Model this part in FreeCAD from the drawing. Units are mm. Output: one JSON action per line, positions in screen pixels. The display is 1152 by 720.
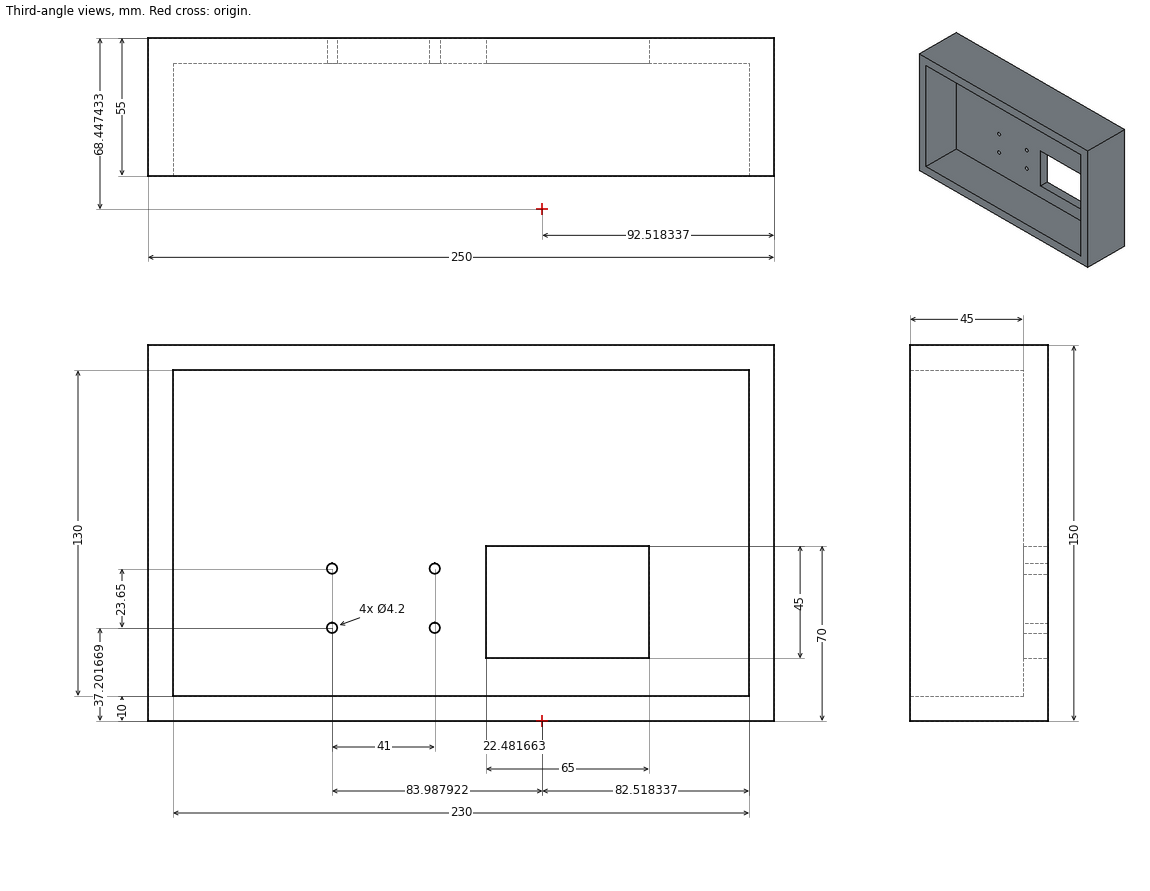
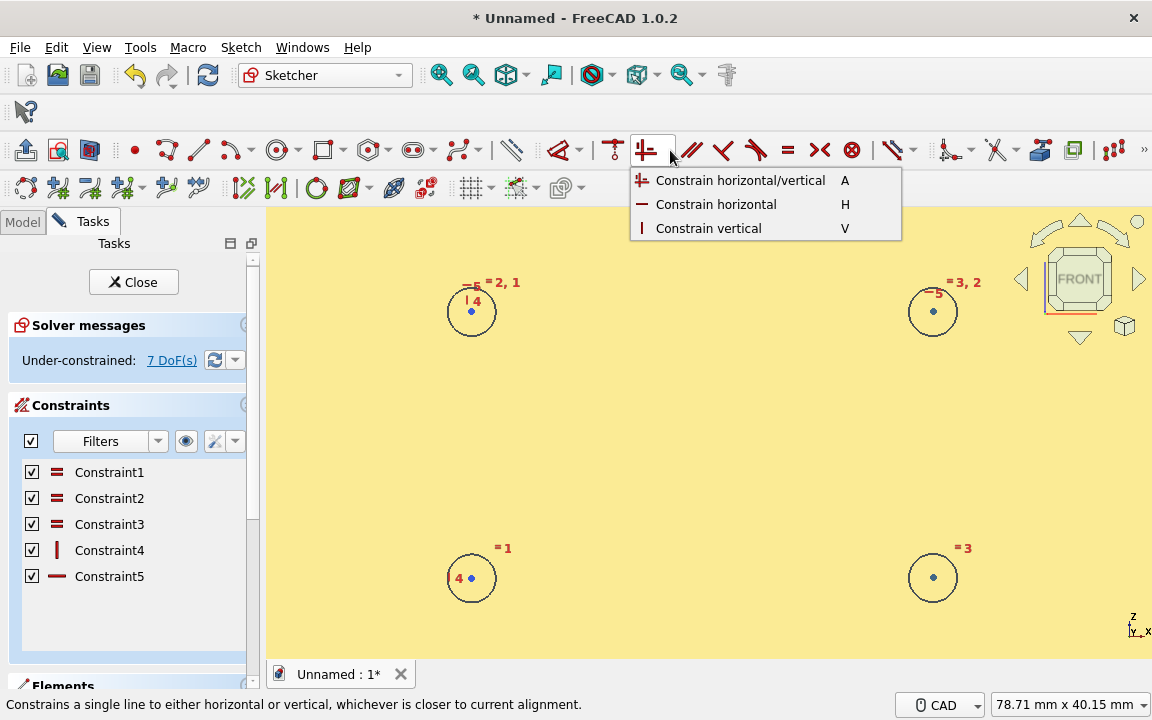
{"action": "left_click", "coordinate": [766, 228]}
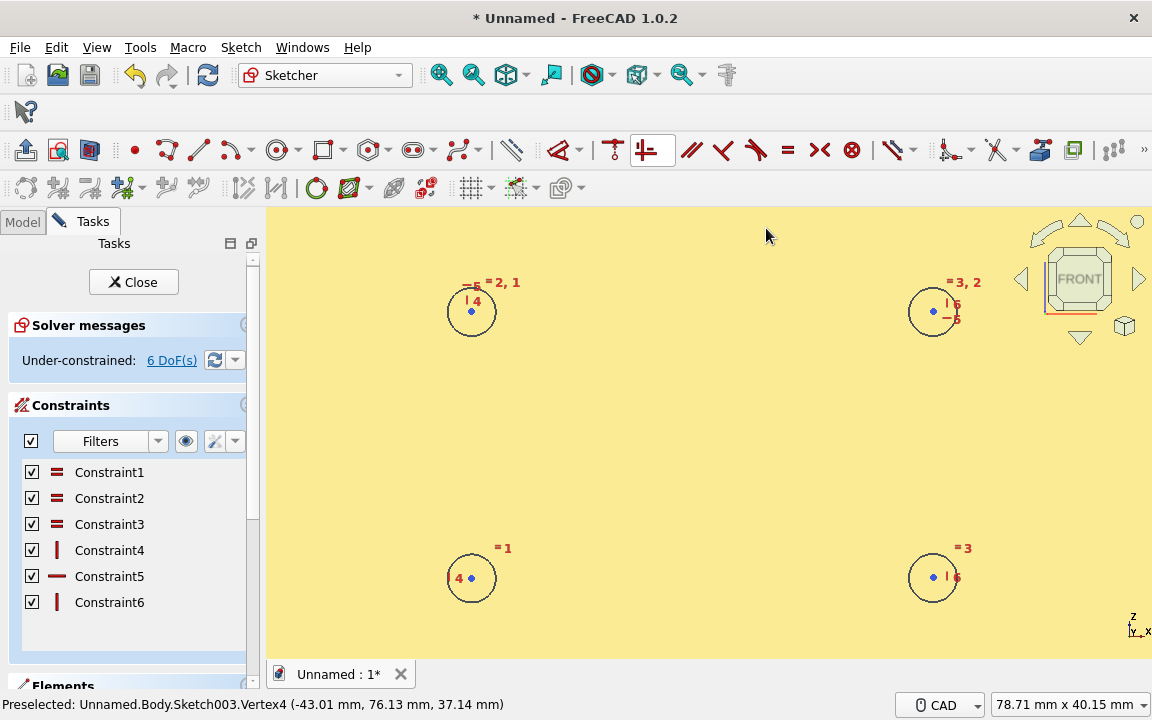
{"action": "left_click", "coordinate": [472, 578]}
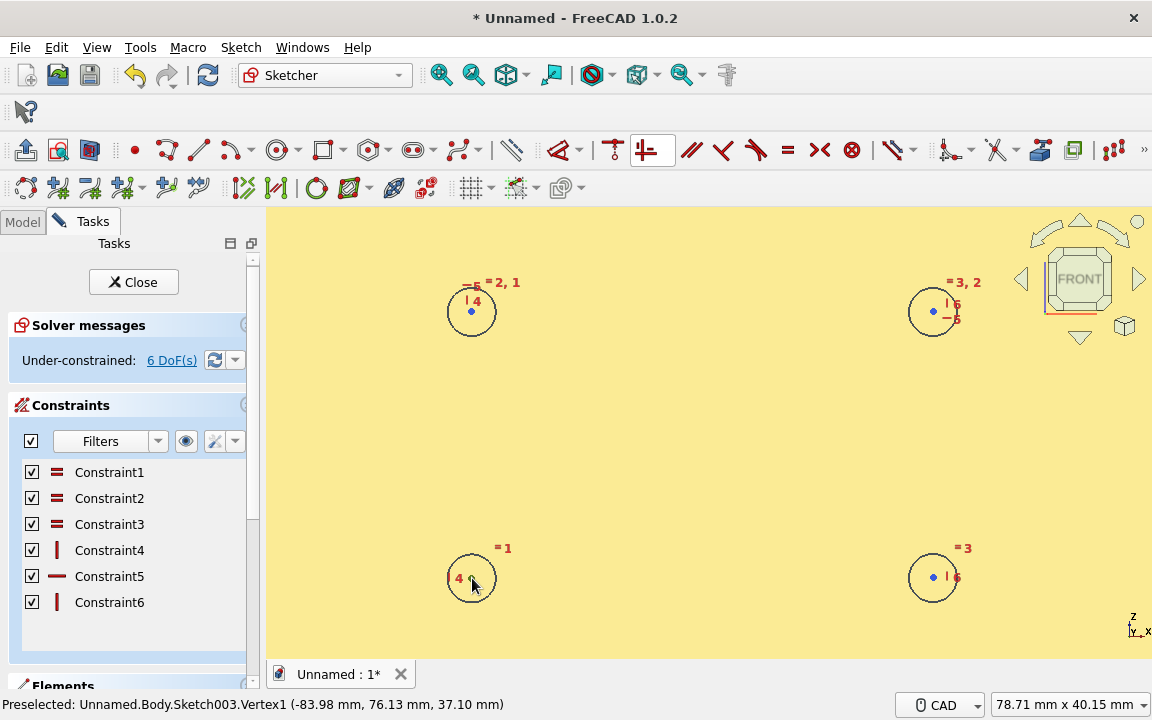
{"action": "left_click", "coordinate": [933, 578]}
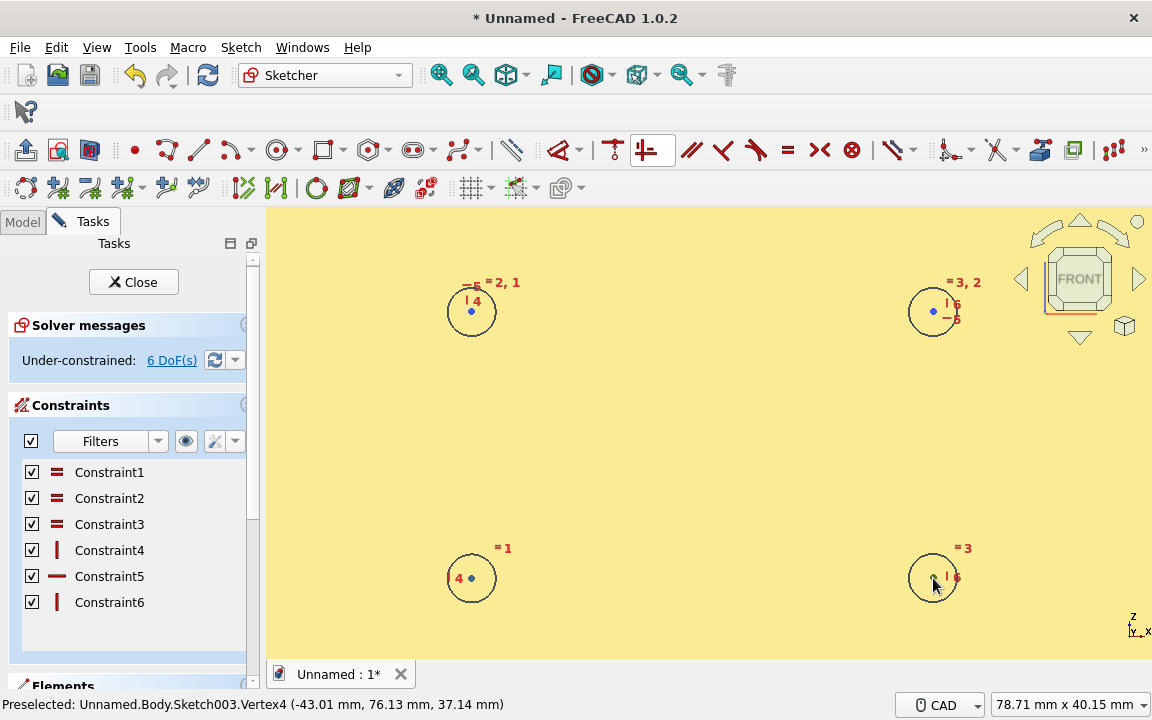
{"action": "left_click", "coordinate": [670, 150]}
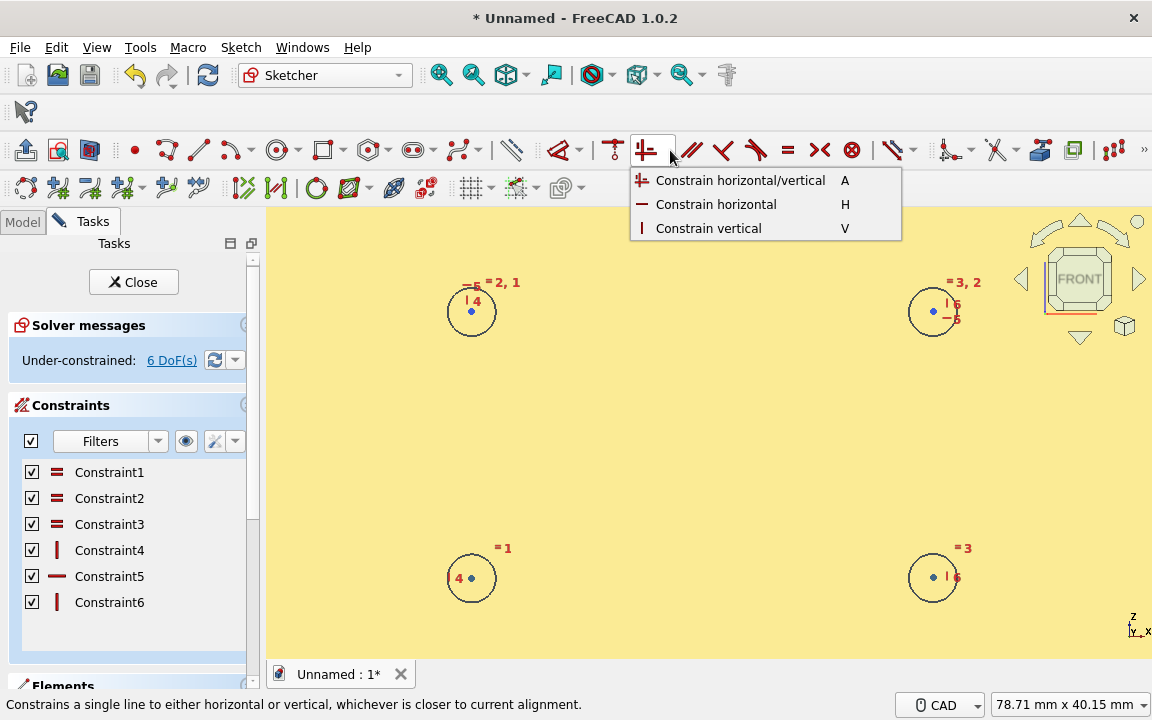
{"action": "left_click", "coordinate": [766, 204]}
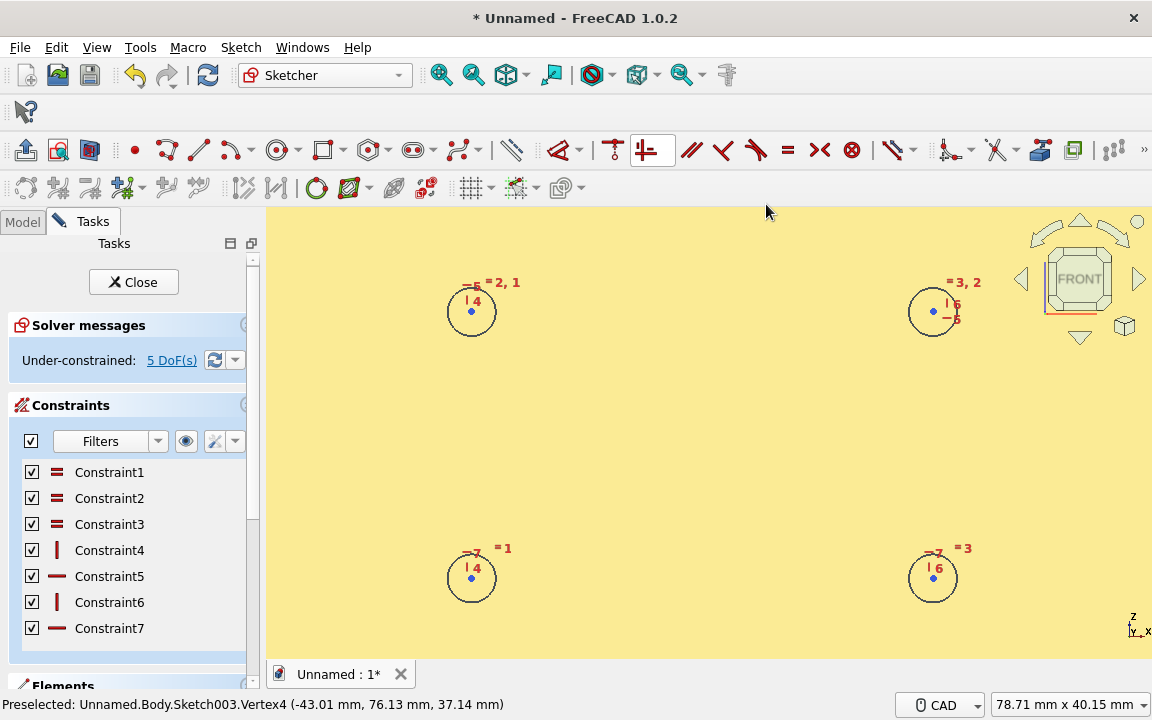
{"action": "left_click", "coordinate": [558, 150]}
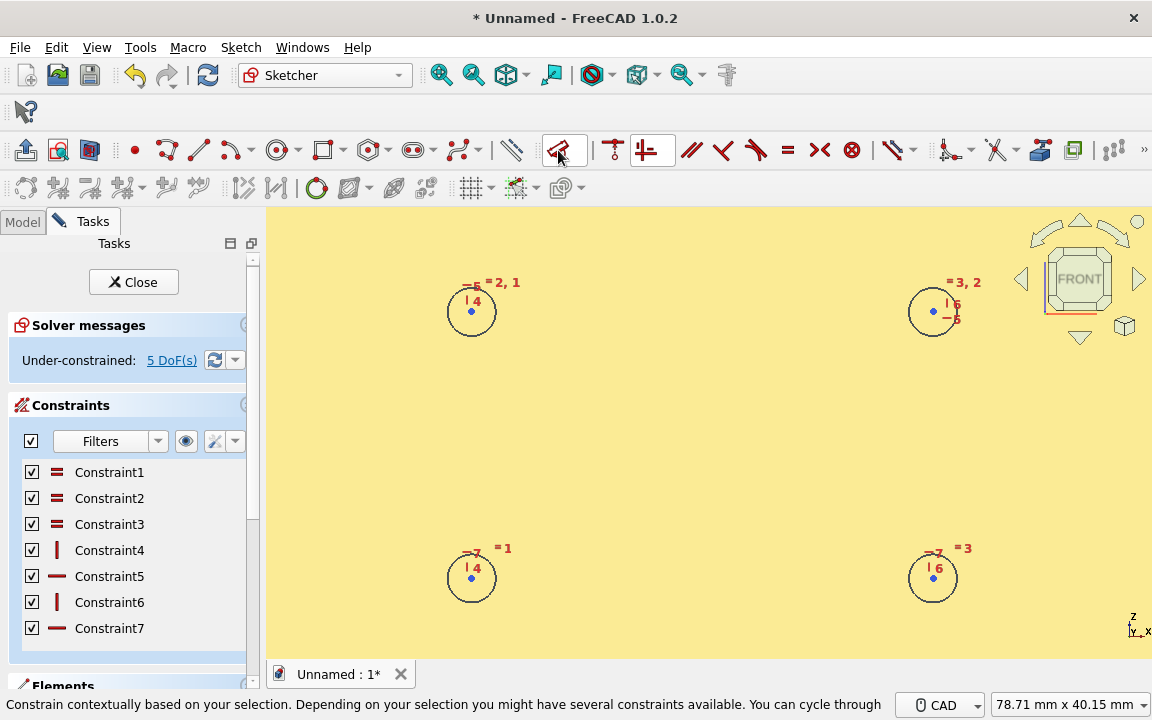
{"action": "left_click", "coordinate": [489, 561]}
{"action": "left_click", "coordinate": [511, 538]}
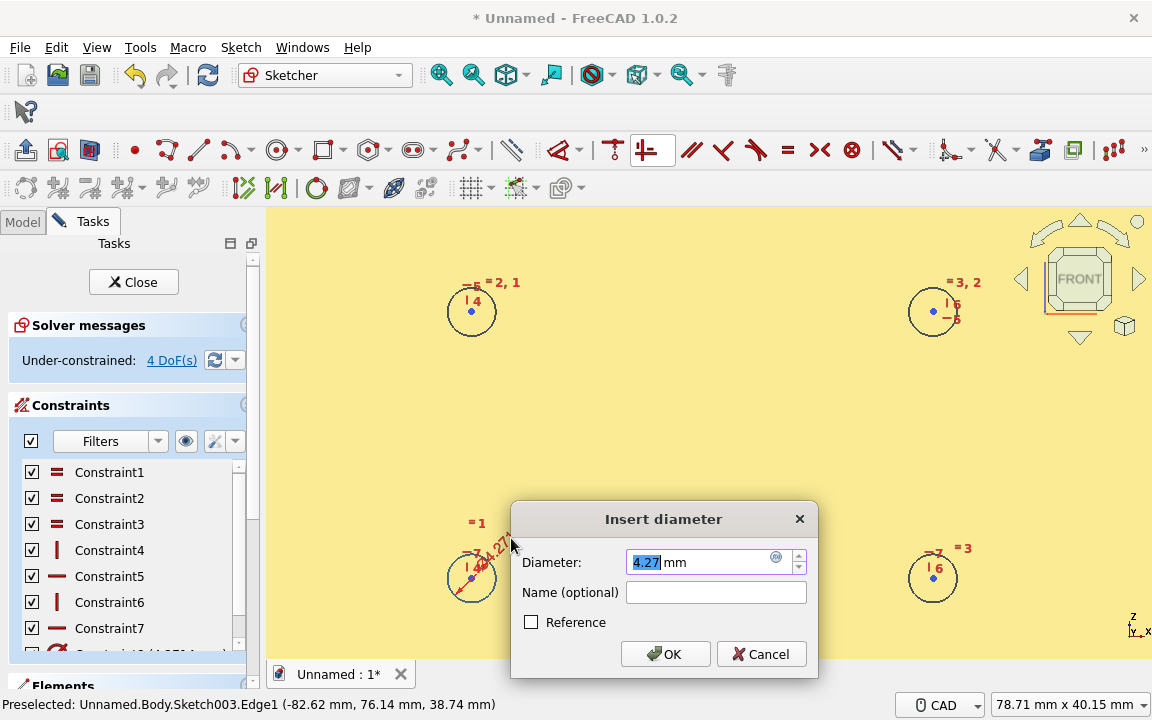
{"action": "type", "text": "4.2"}
{"action": "key", "text": "Return"}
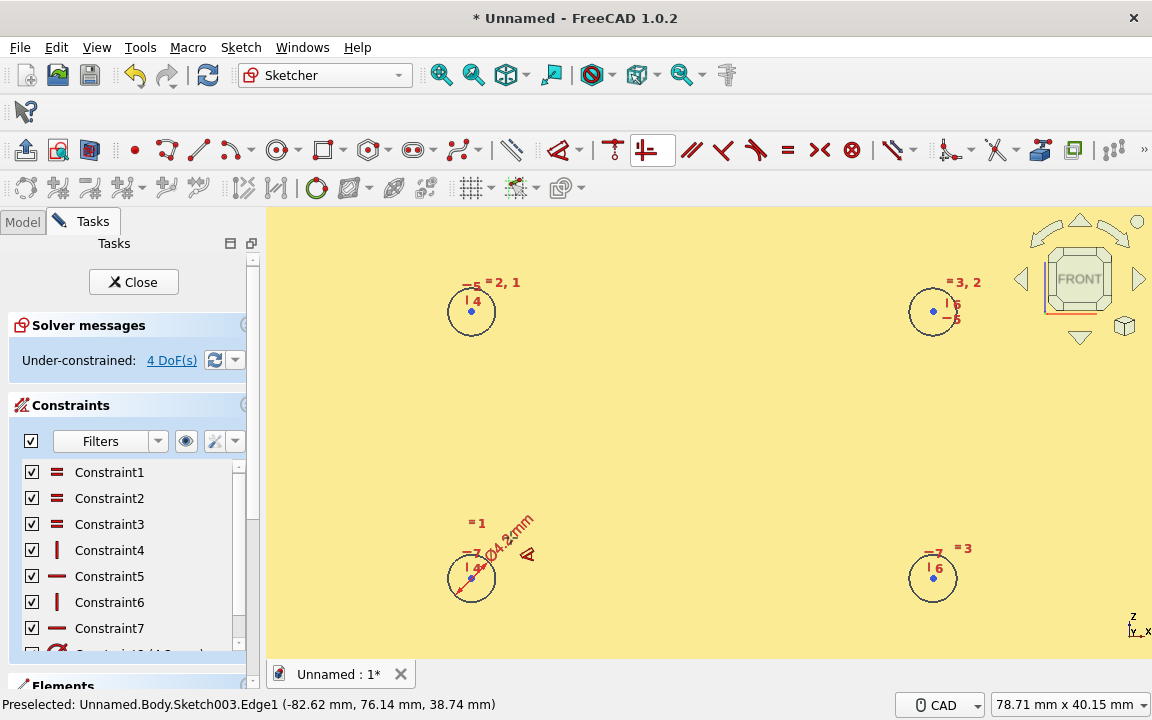
{"action": "left_click", "coordinate": [472, 312]}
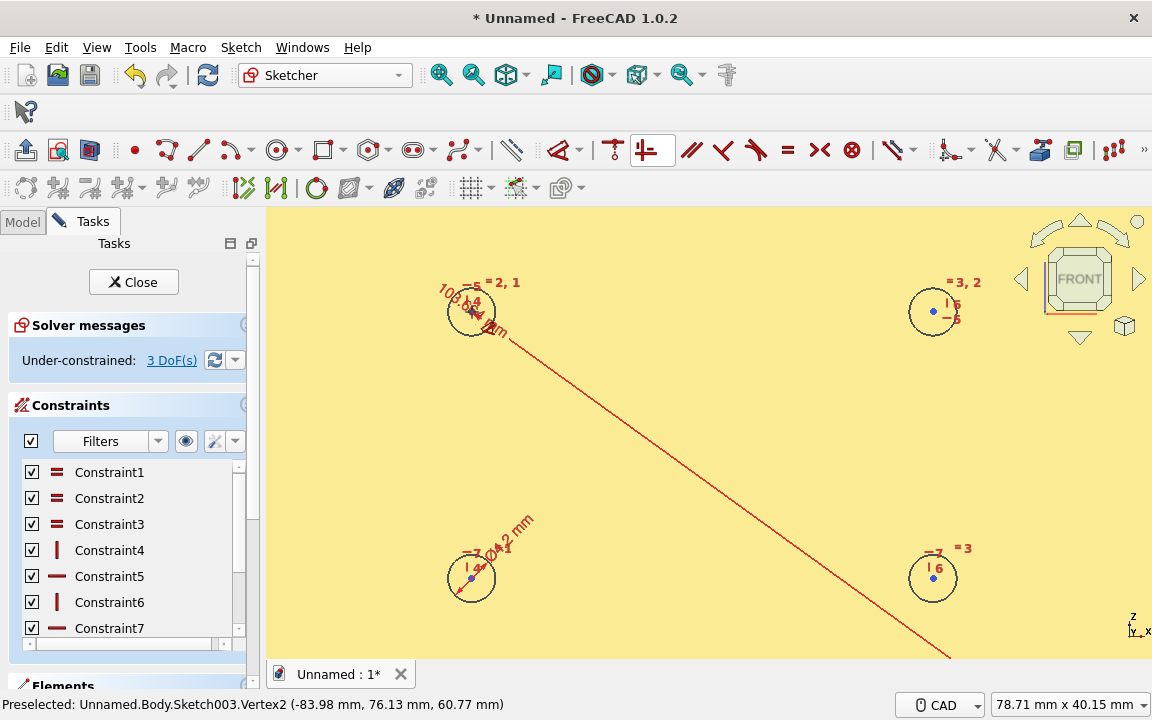
{"action": "left_click", "coordinate": [933, 312]}
{"action": "left_click", "coordinate": [702, 278]}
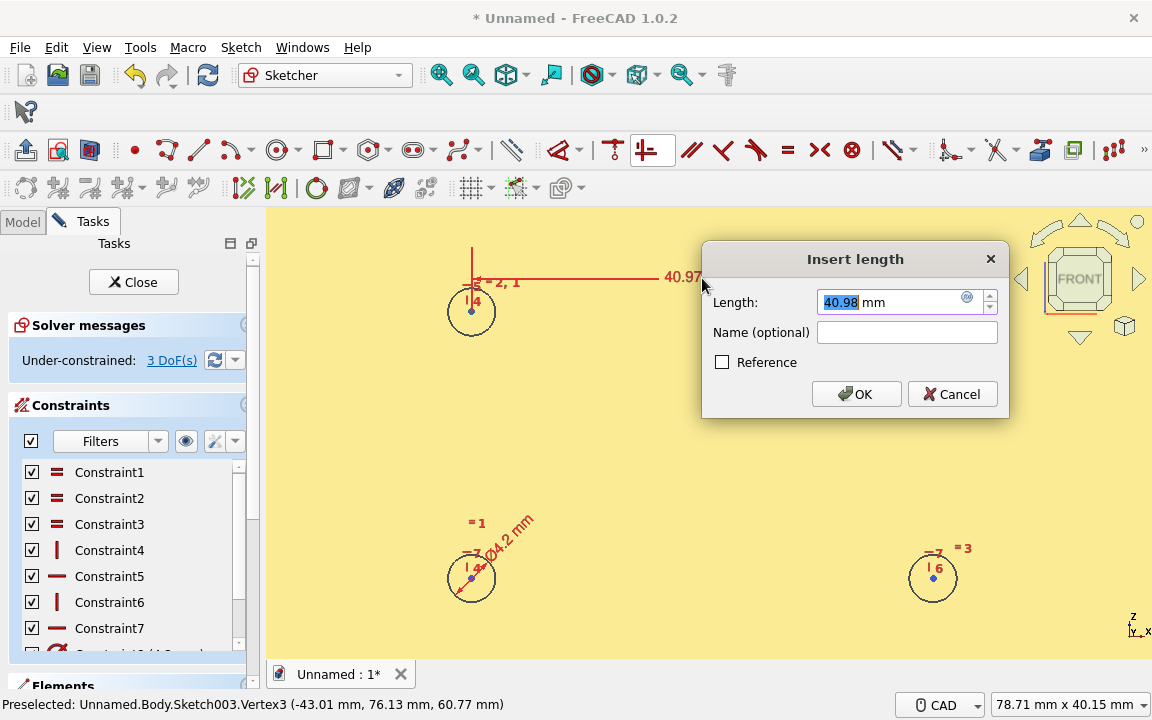
{"action": "type", "text": "41"}
{"action": "key", "text": "Return"}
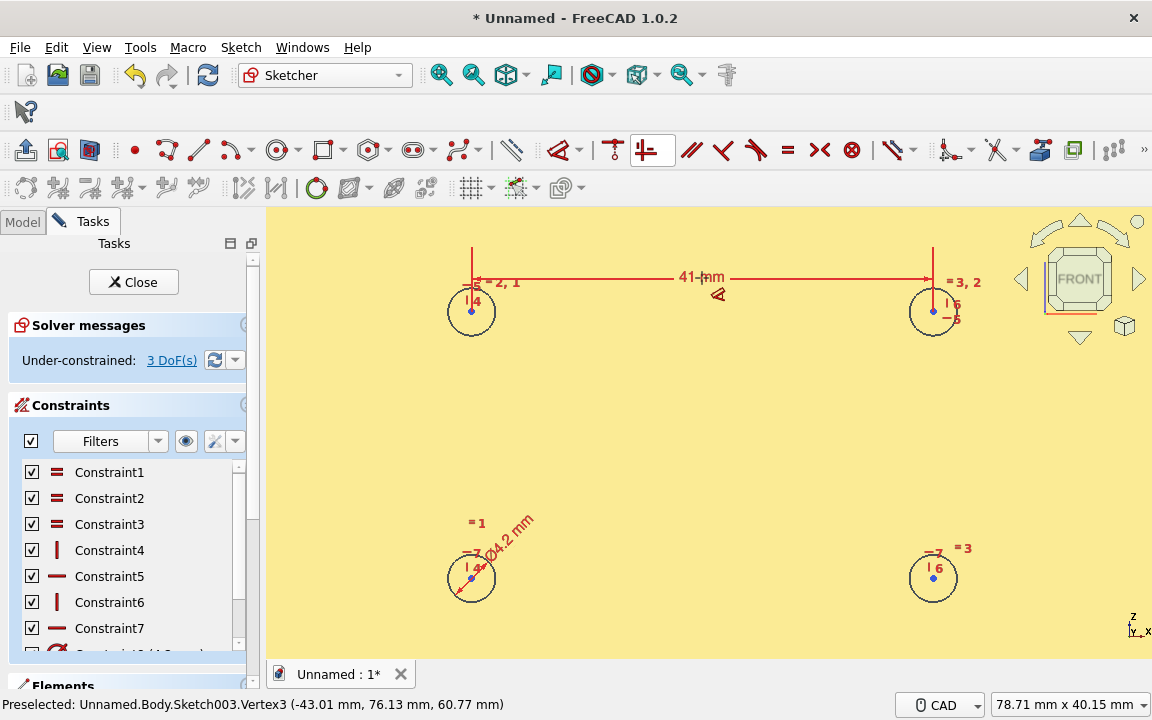
{"action": "left_click", "coordinate": [472, 578]}